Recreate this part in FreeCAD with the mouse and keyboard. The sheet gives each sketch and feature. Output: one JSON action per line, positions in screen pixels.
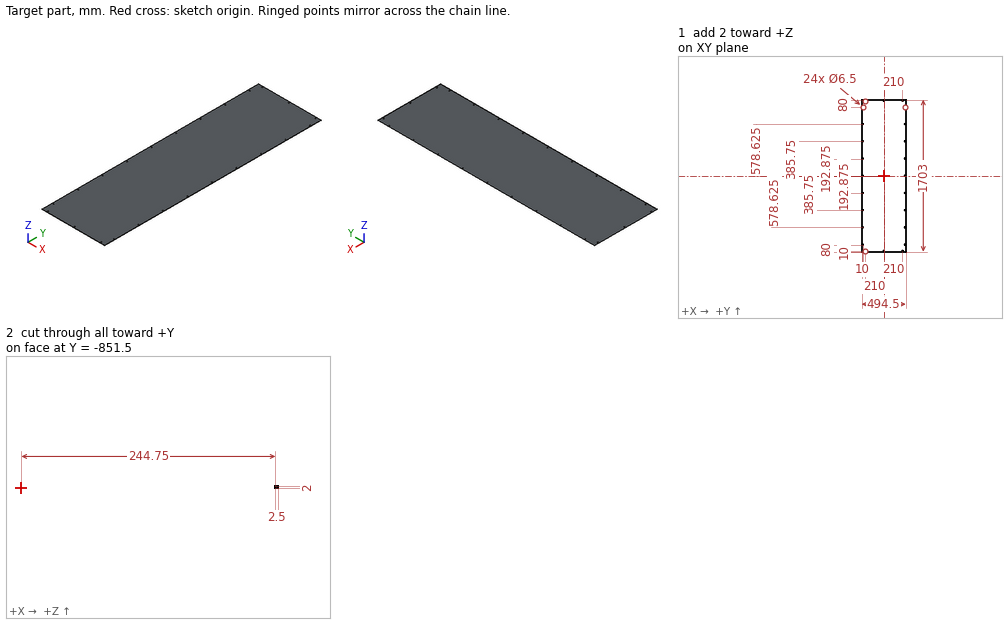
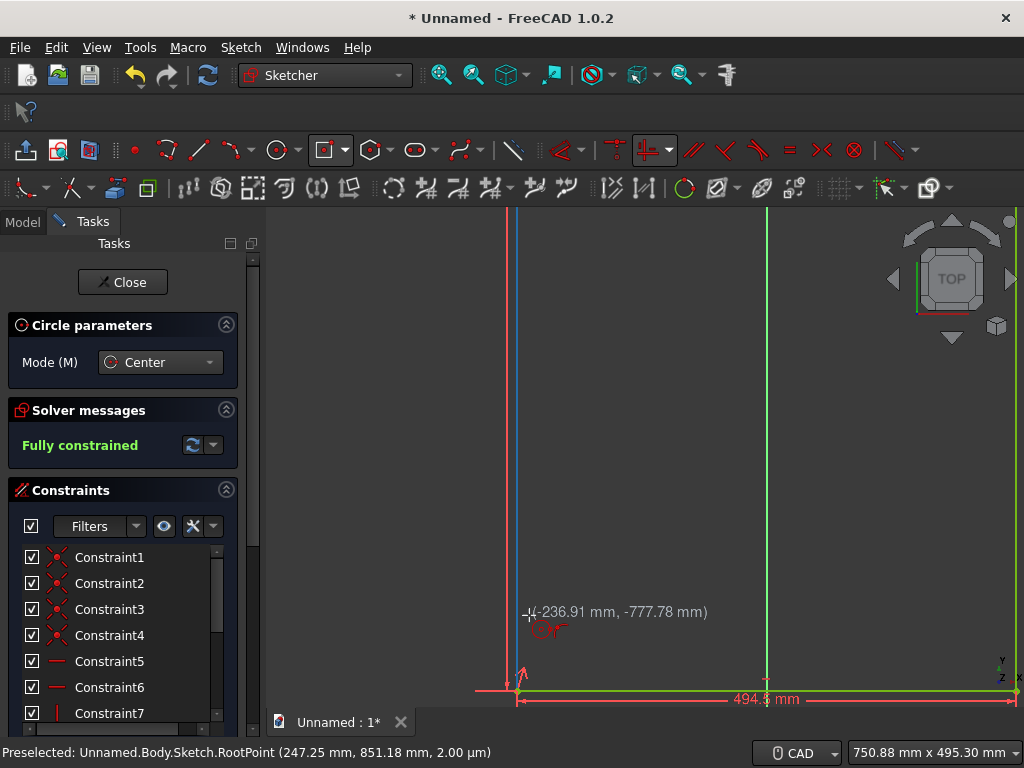
{"action": "left_click", "coordinate": [526, 606]}
{"action": "mouse_move", "coordinate": [530, 602]}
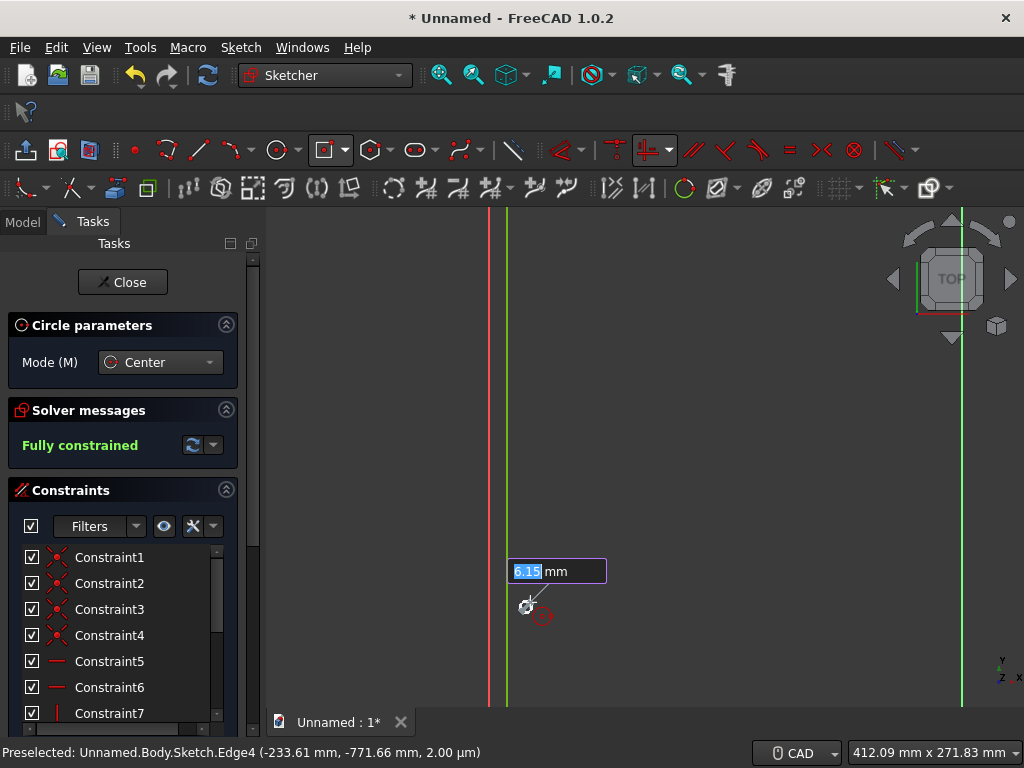
{"action": "type", "text": "6.5"}
{"action": "key", "text": "Return"}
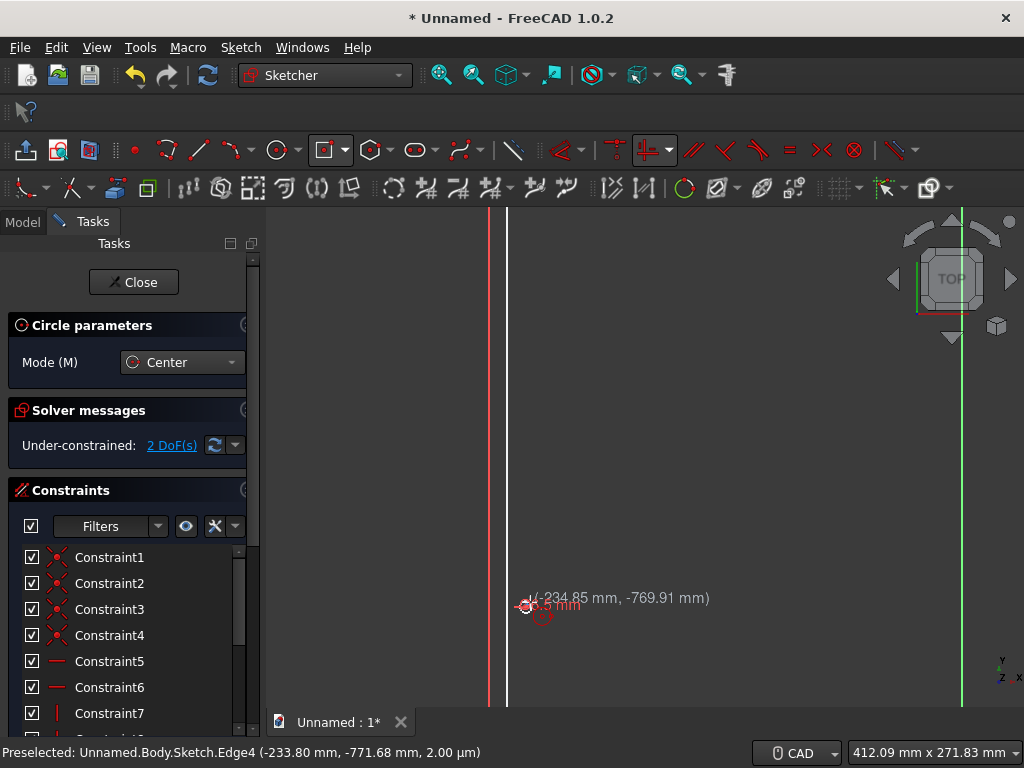
{"action": "scroll", "coordinate": [538, 584], "scroll_direction": "down", "scroll_amount": 12}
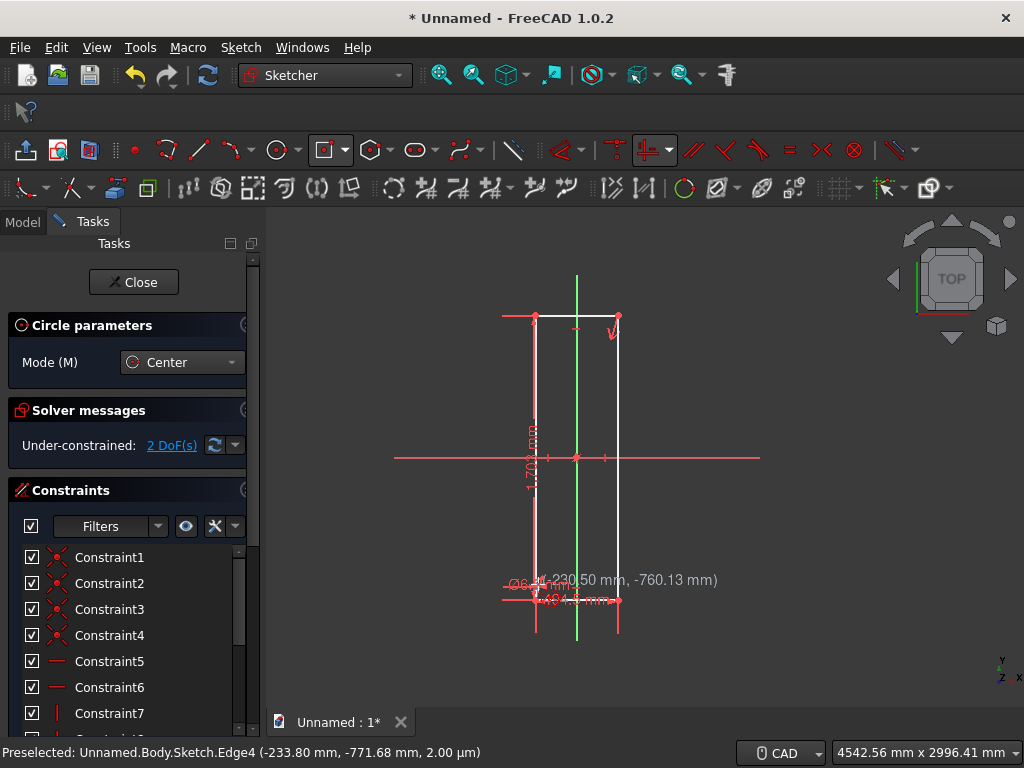
{"action": "scroll", "coordinate": [542, 598], "scroll_direction": "up", "scroll_amount": 19}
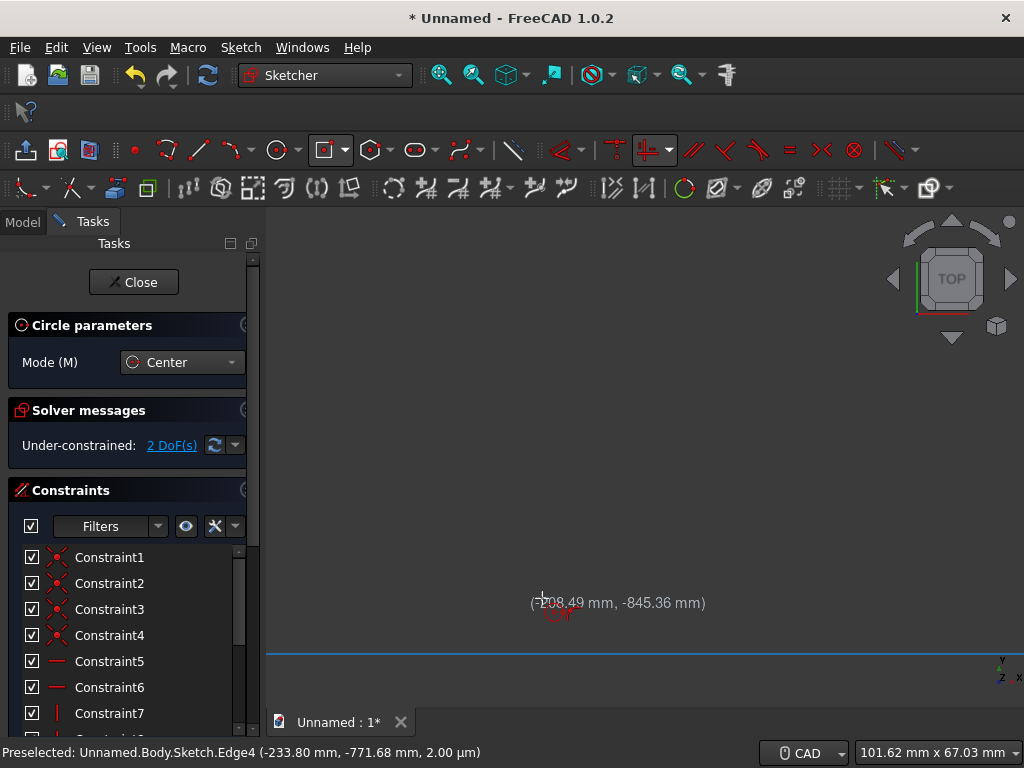
{"action": "scroll", "coordinate": [534, 630], "scroll_direction": "down", "scroll_amount": 18}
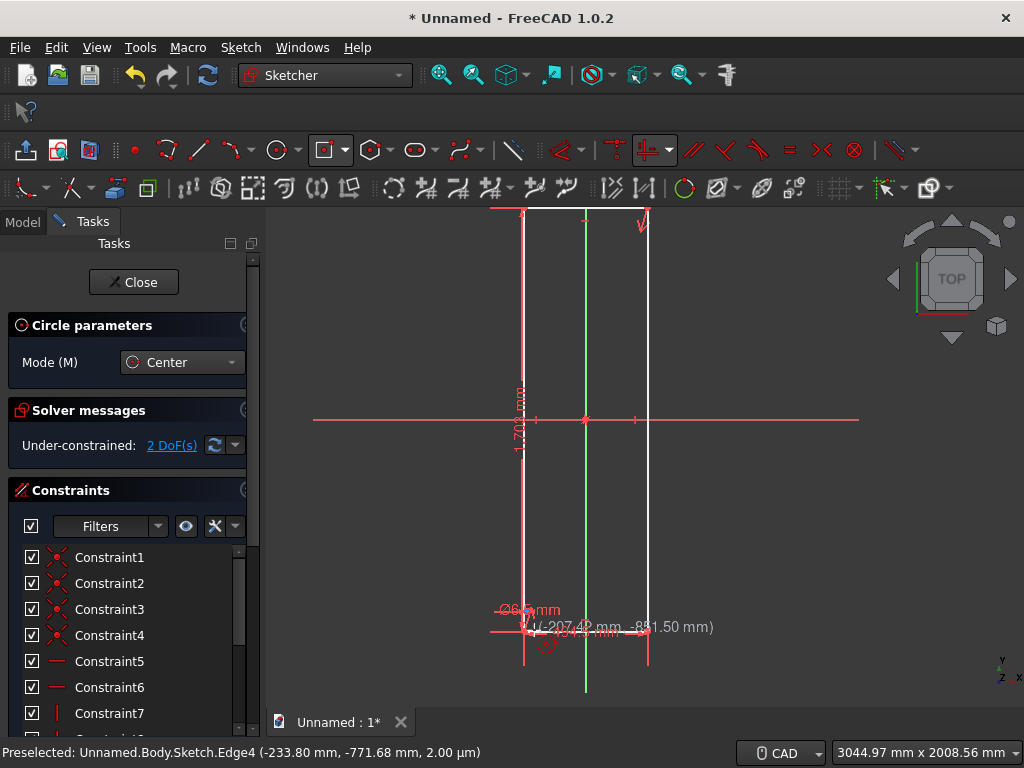
{"action": "scroll", "coordinate": [534, 629], "scroll_direction": "up", "scroll_amount": 11}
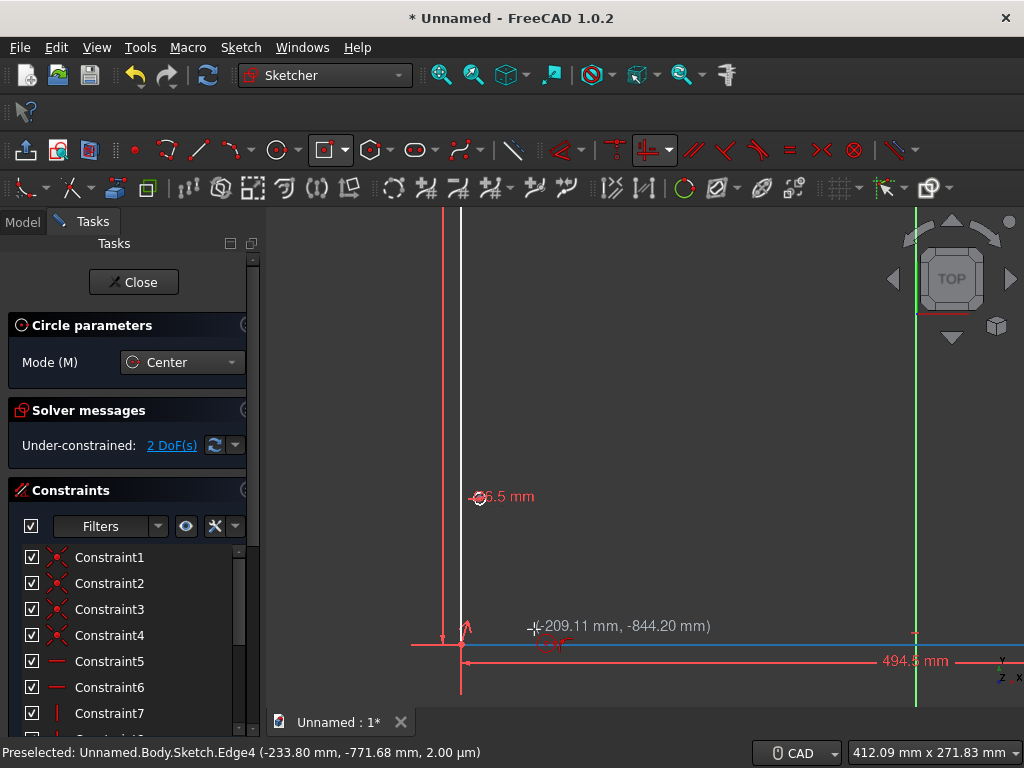
{"action": "left_click", "coordinate": [530, 626]}
{"action": "mouse_move", "coordinate": [534, 622]}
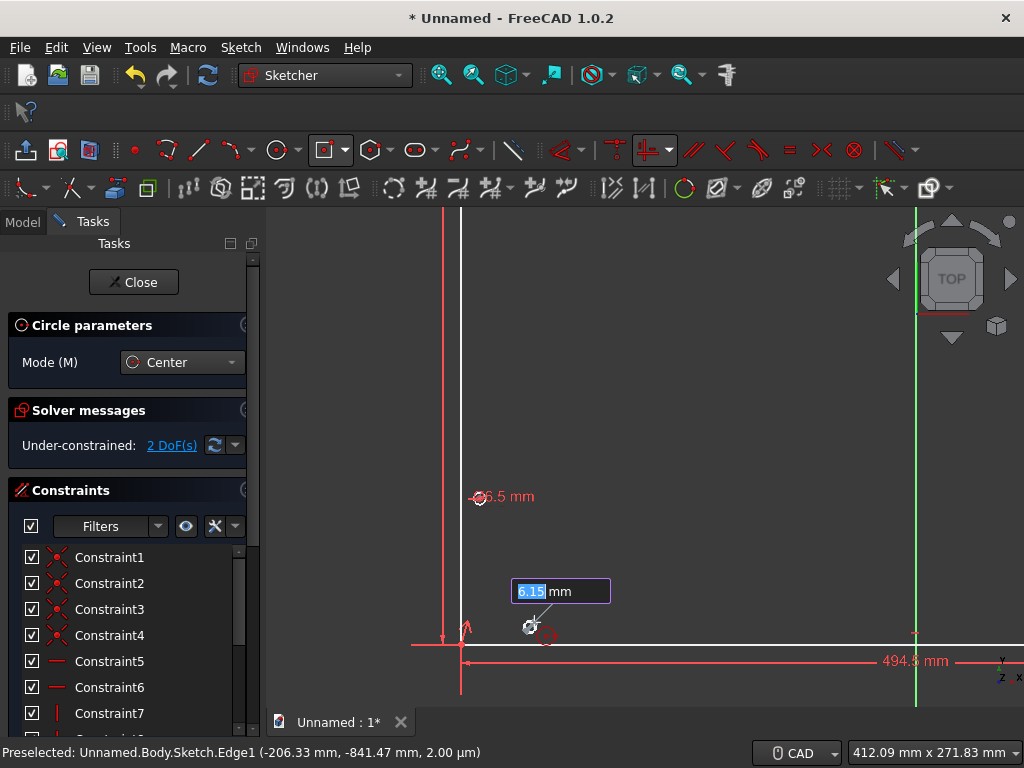
{"action": "type", "text": "6.5"}
{"action": "key", "text": "Return"}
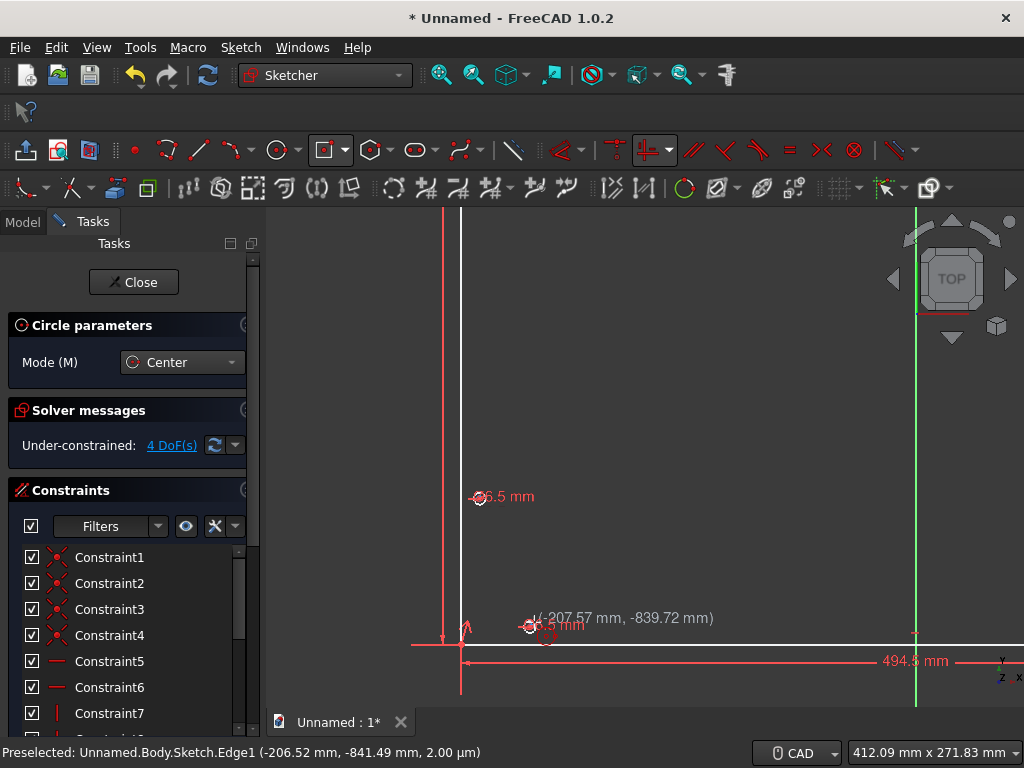
{"action": "scroll", "coordinate": [543, 595], "scroll_direction": "down", "scroll_amount": 12}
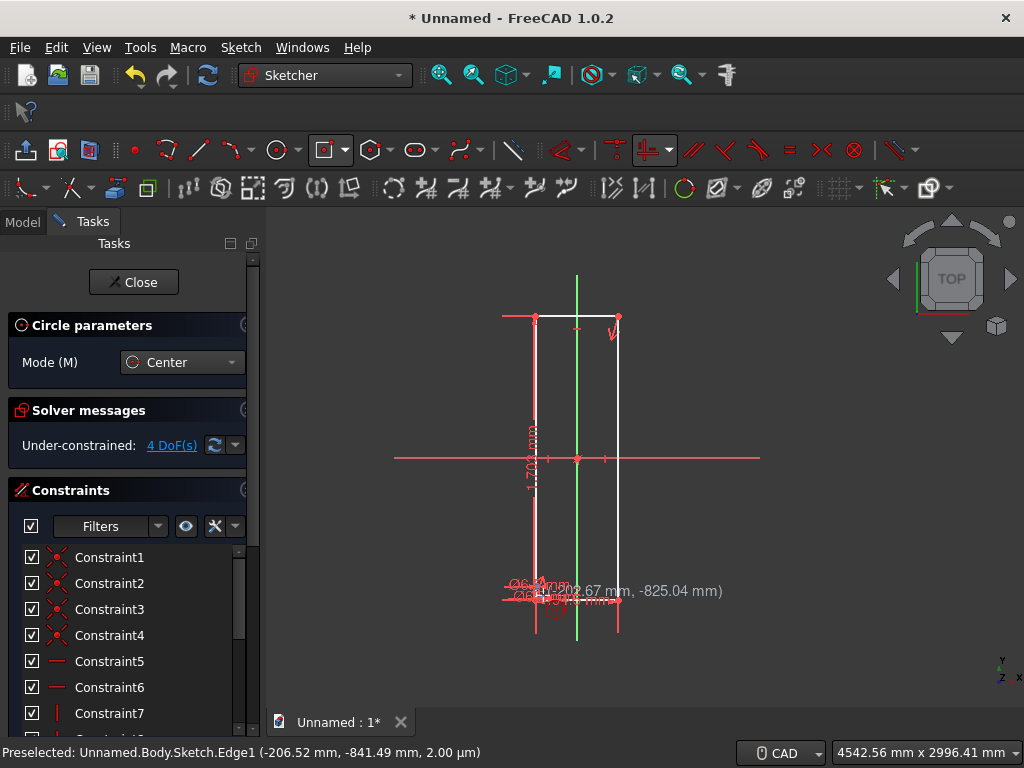
{"action": "scroll", "coordinate": [538, 555], "scroll_direction": "up", "scroll_amount": 19}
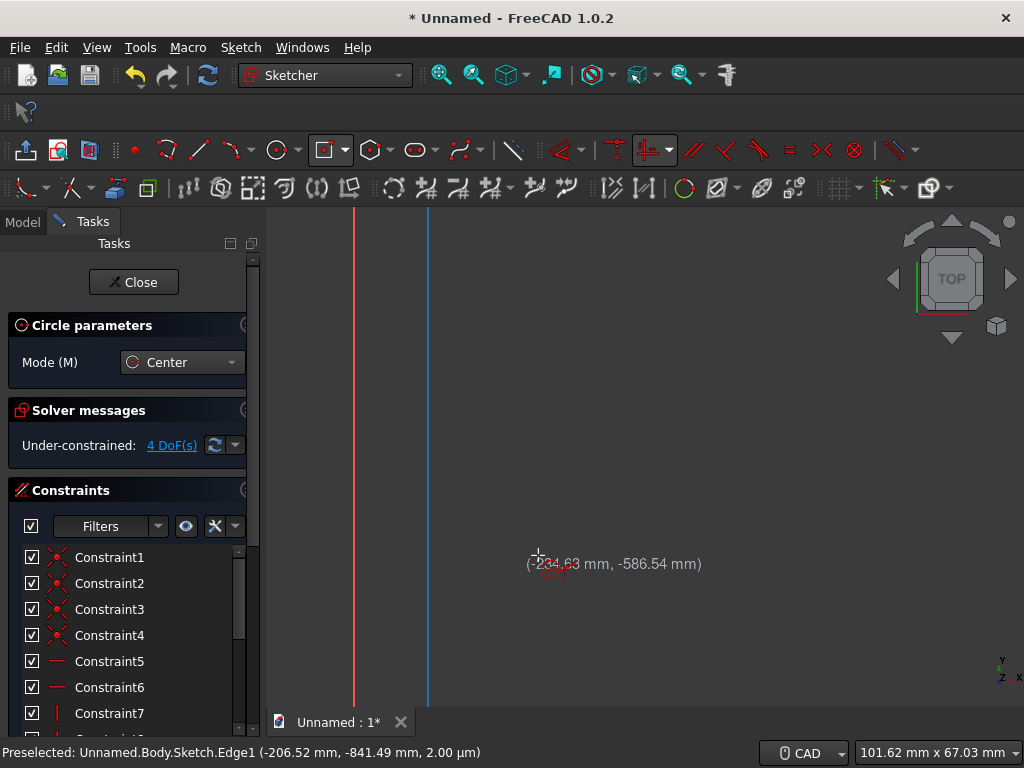
{"action": "scroll", "coordinate": [529, 577], "scroll_direction": "down", "scroll_amount": 18}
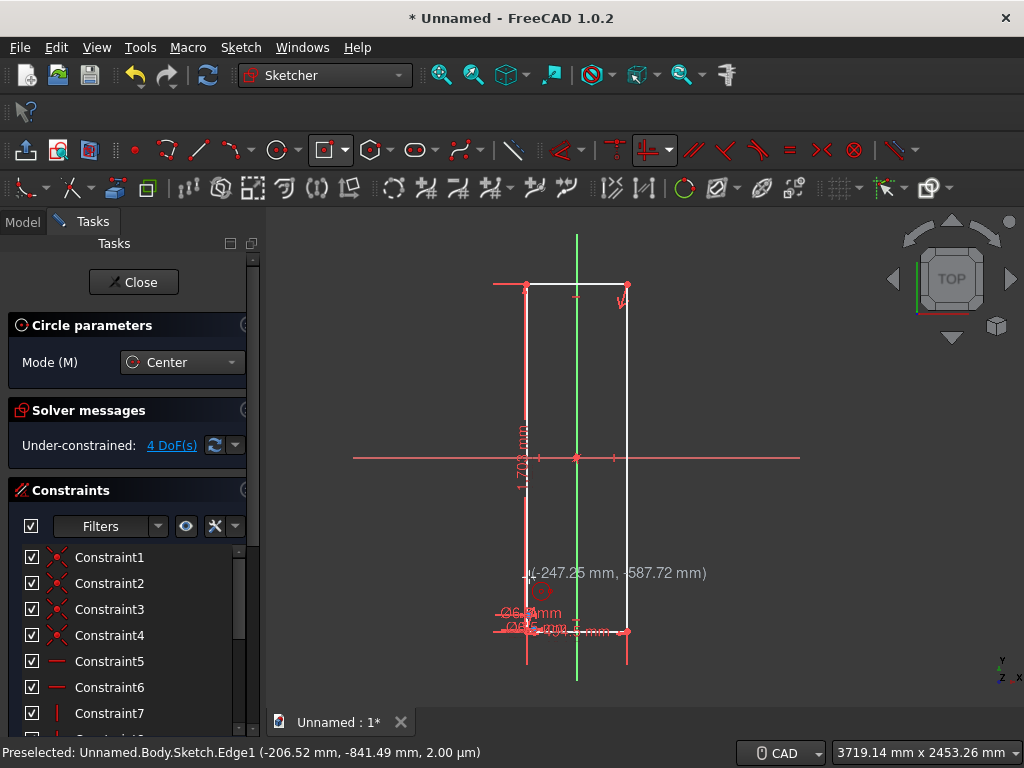
{"action": "scroll", "coordinate": [529, 576], "scroll_direction": "up", "scroll_amount": 11}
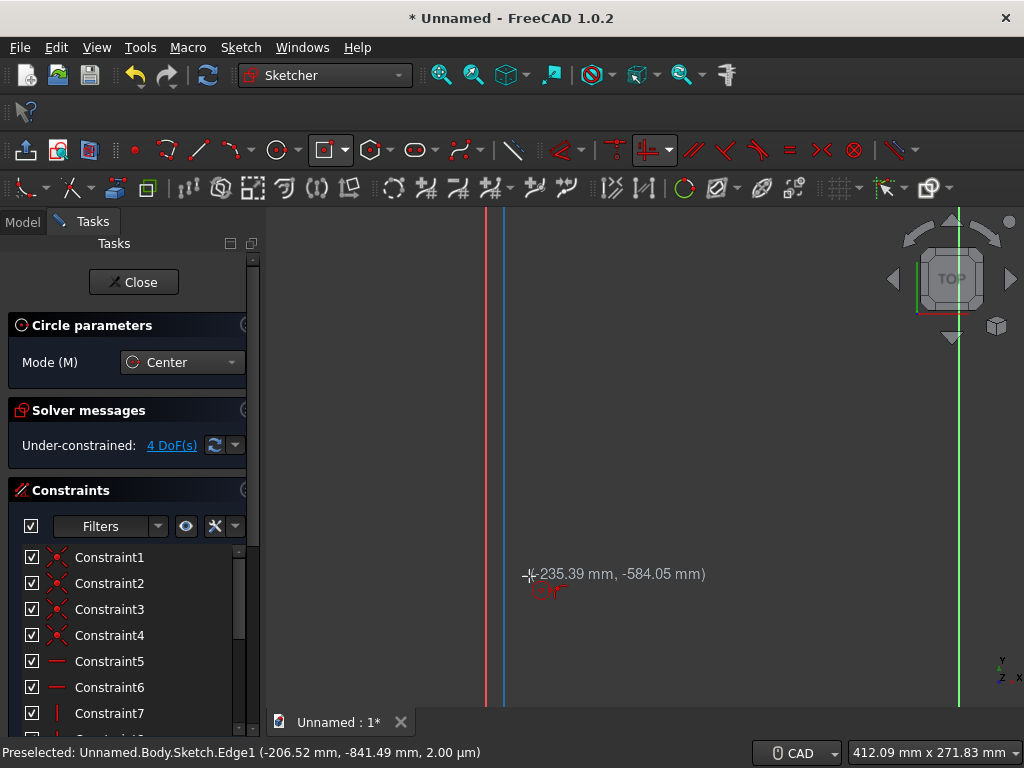
{"action": "left_click", "coordinate": [523, 569]}
{"action": "mouse_move", "coordinate": [527, 565]}